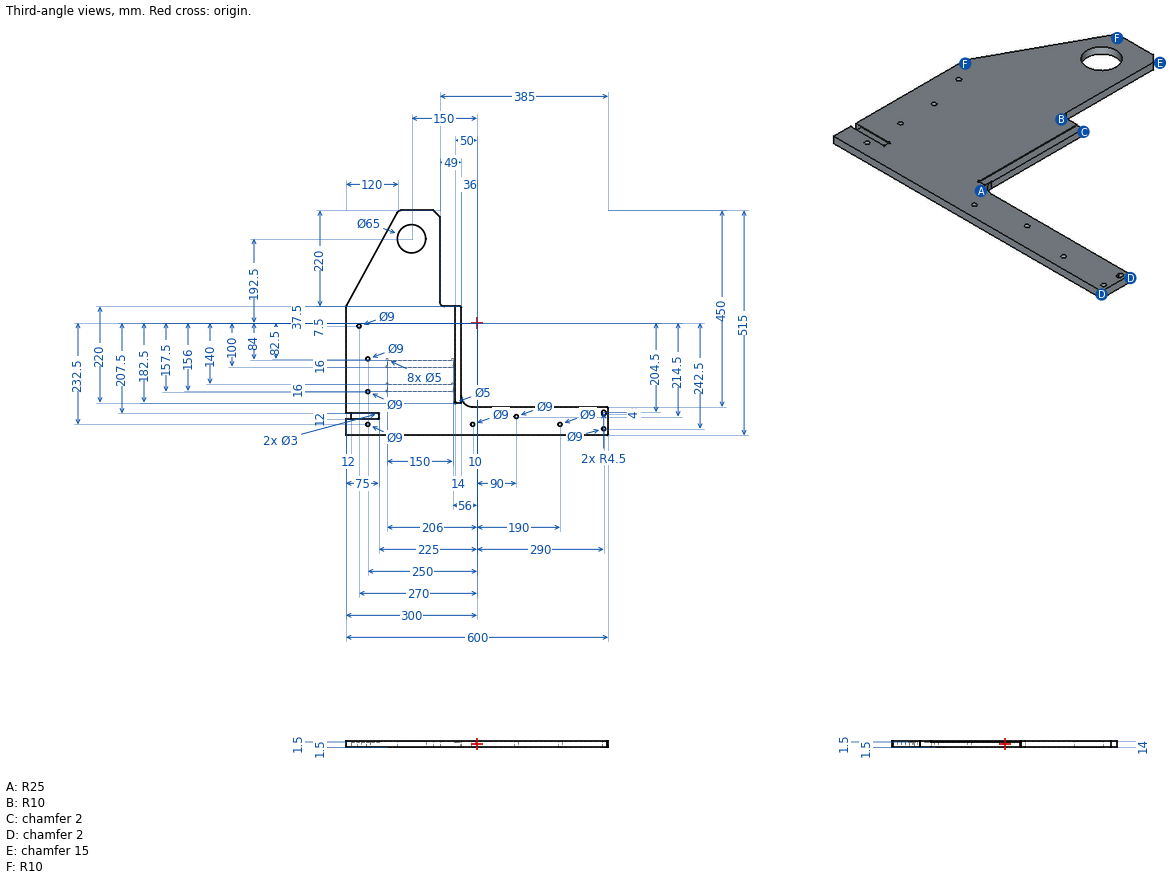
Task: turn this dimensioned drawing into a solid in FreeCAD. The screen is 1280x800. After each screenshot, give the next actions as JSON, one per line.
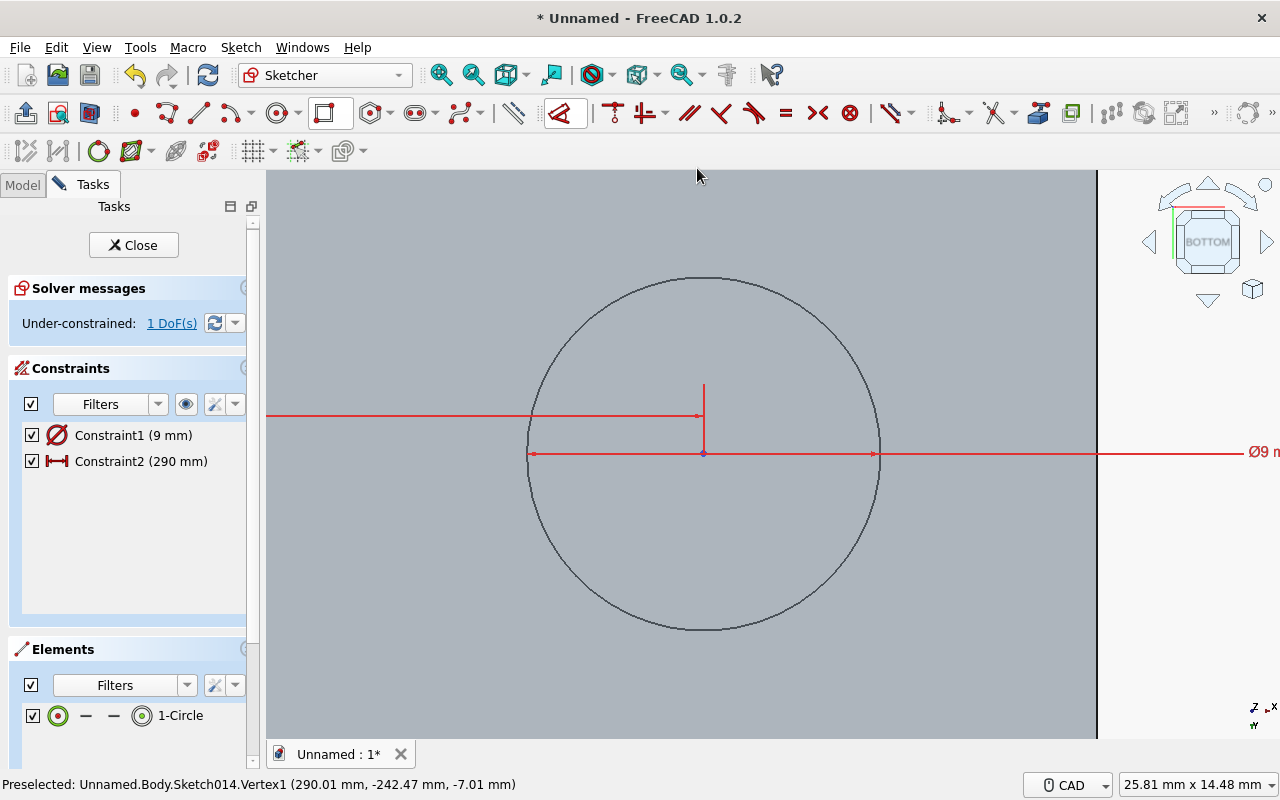
{"action": "left_click", "coordinate": [704, 454]}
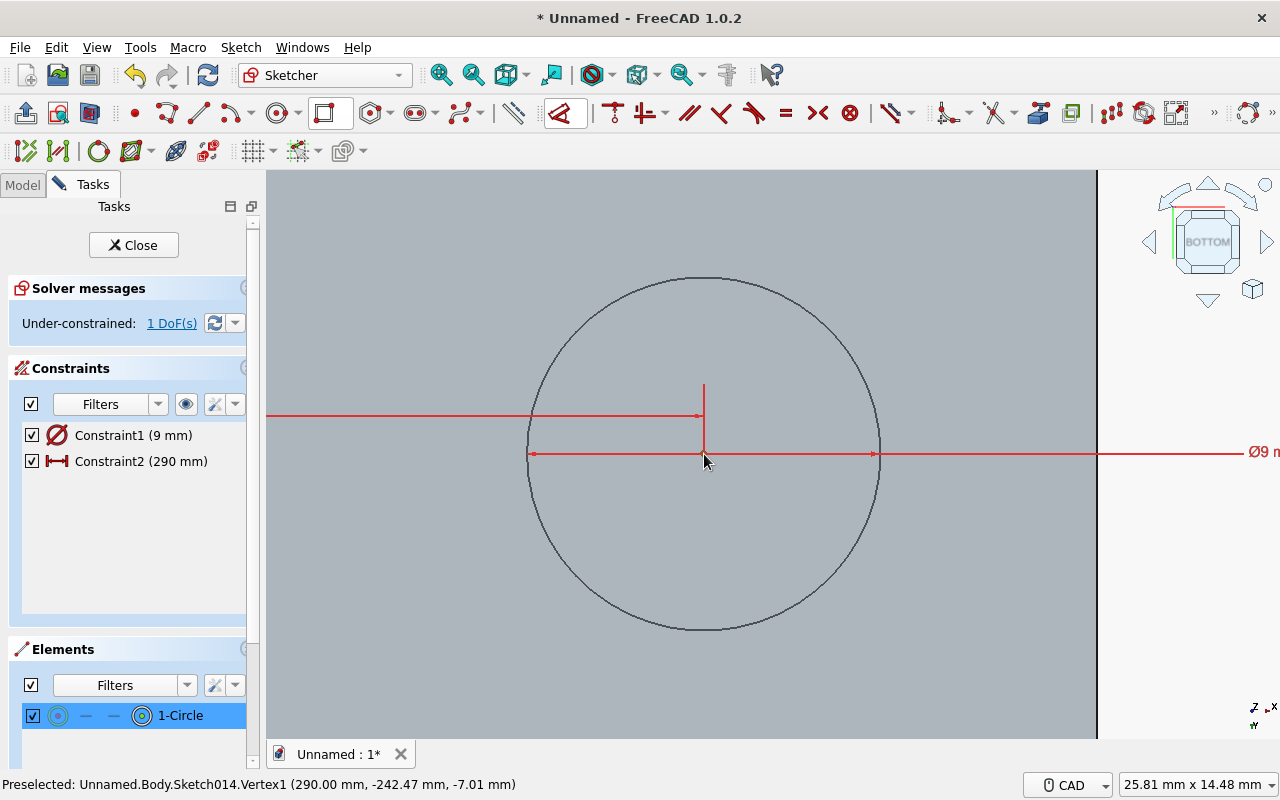
{"action": "left_click", "coordinate": [582, 114]}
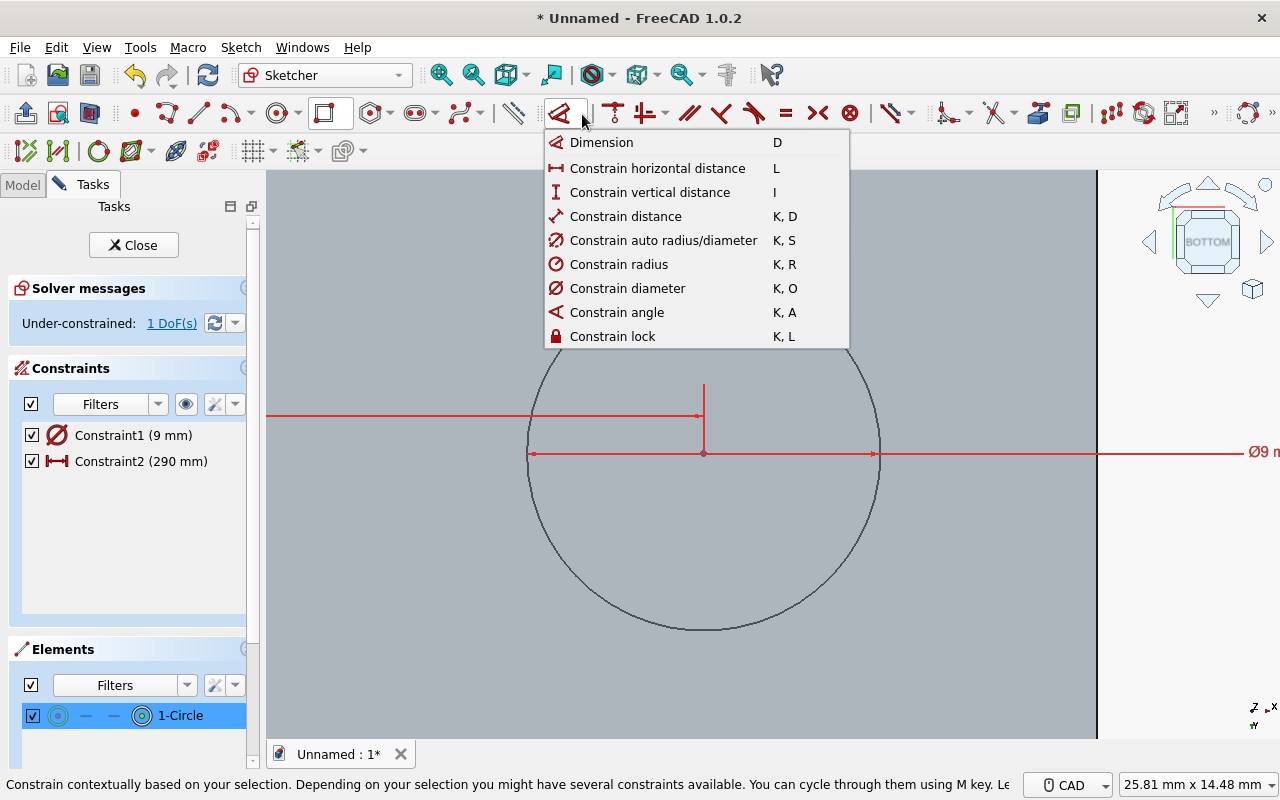
{"action": "left_click", "coordinate": [697, 192]}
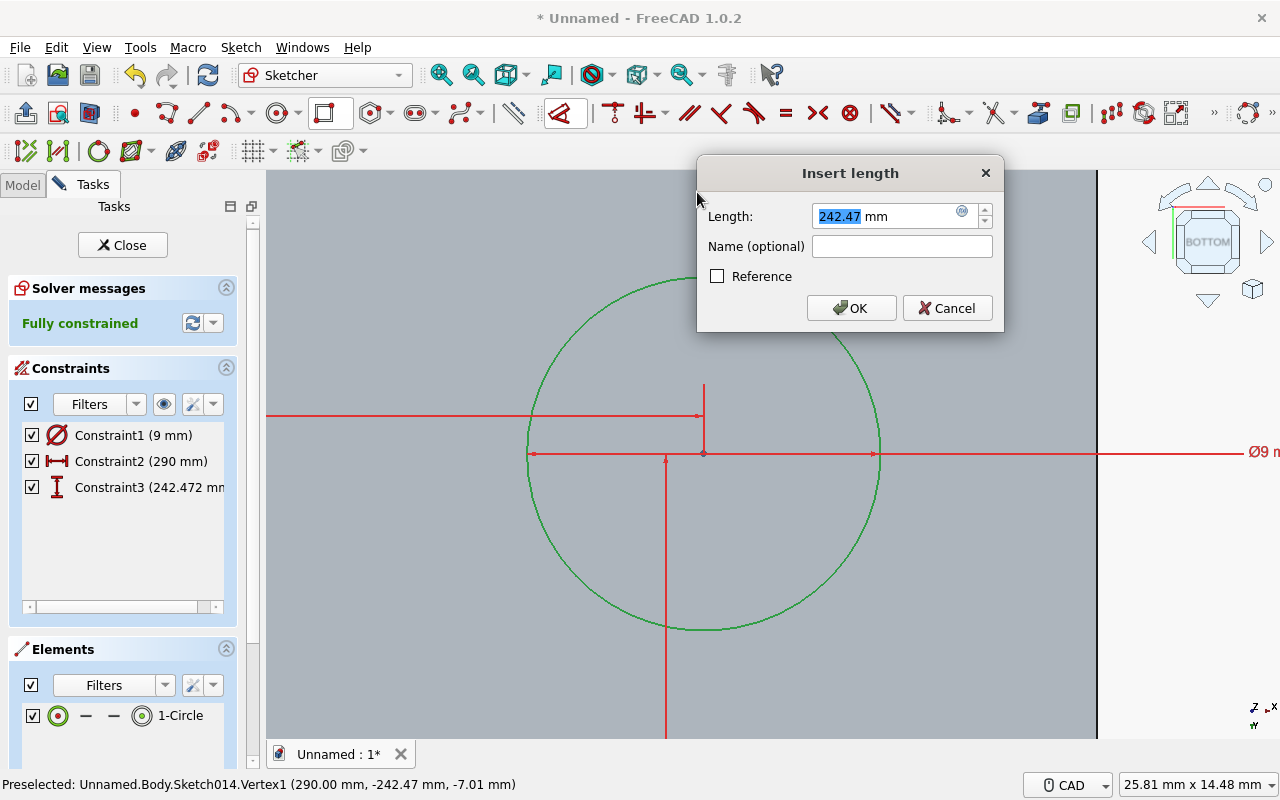
{"action": "type", "text": "242.5"}
{"action": "key", "text": "Return"}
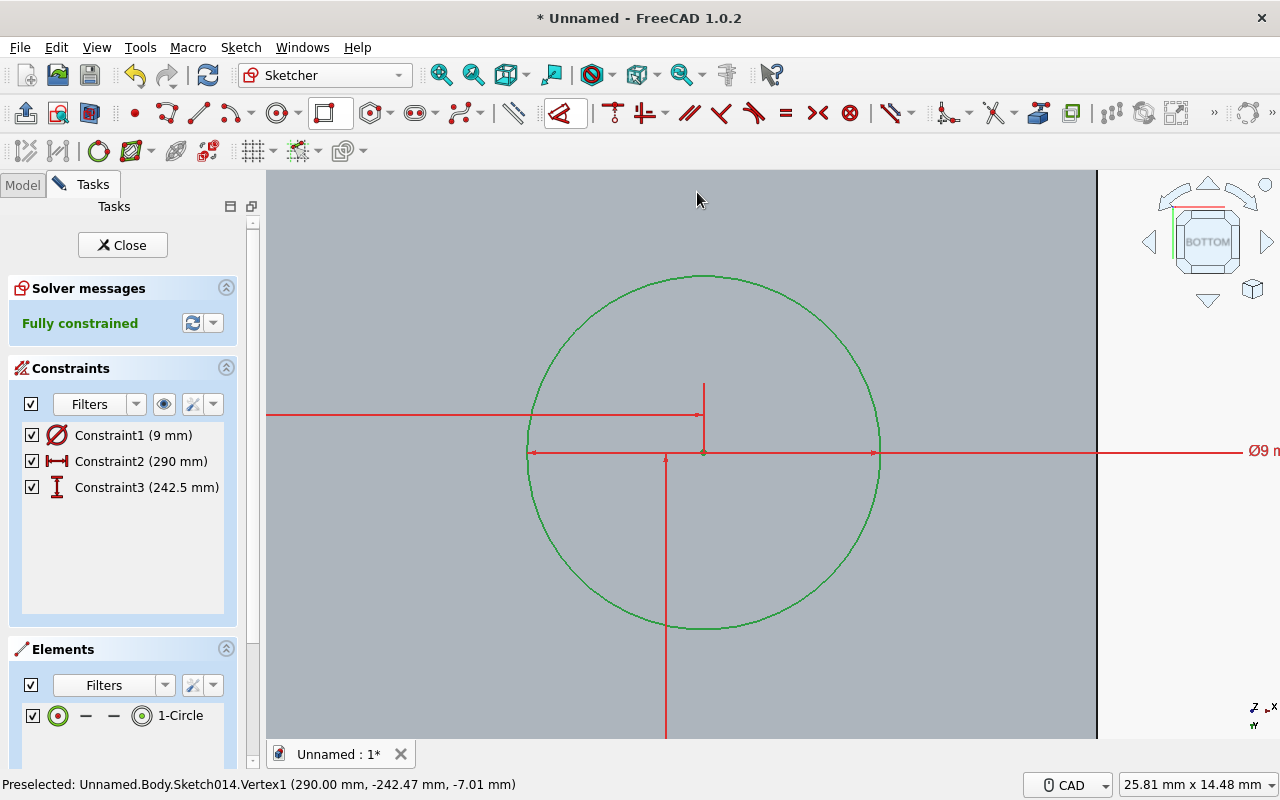
{"action": "left_click", "coordinate": [123, 245]}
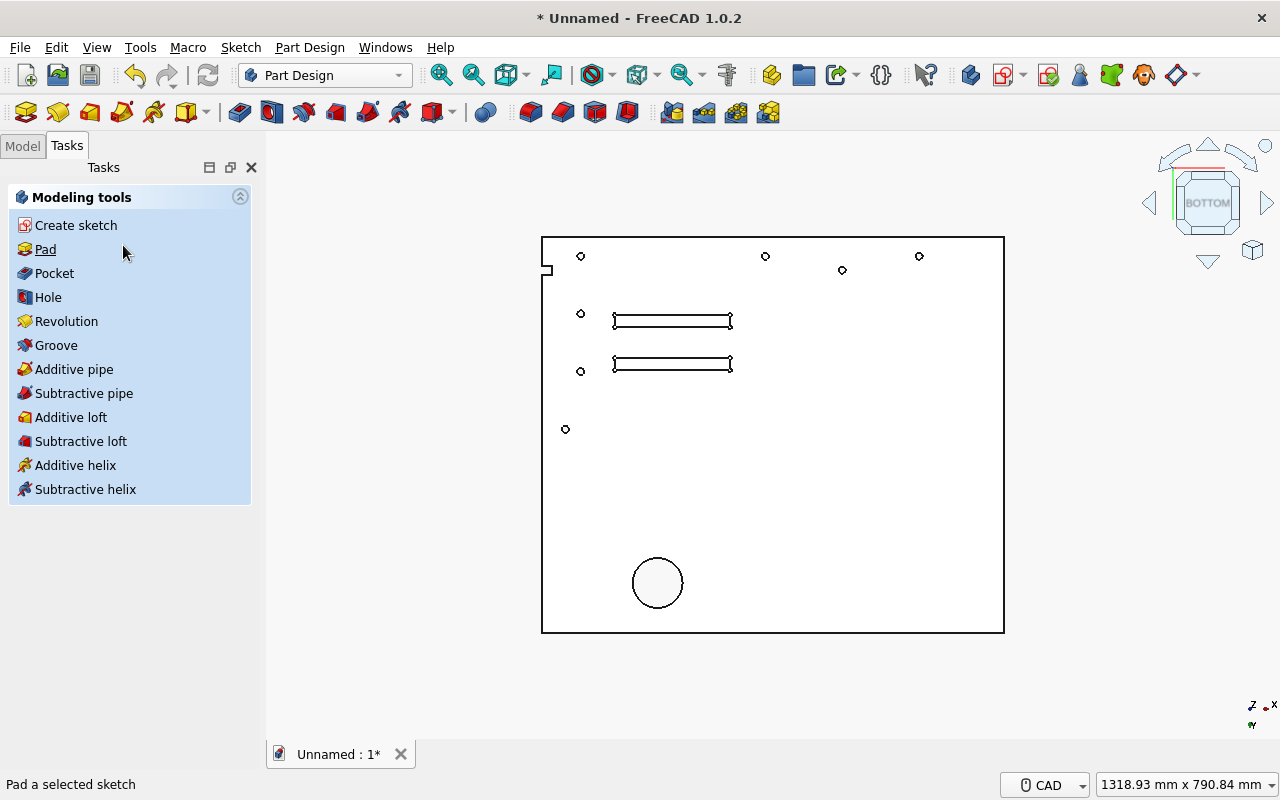
{"action": "left_click", "coordinate": [240, 112]}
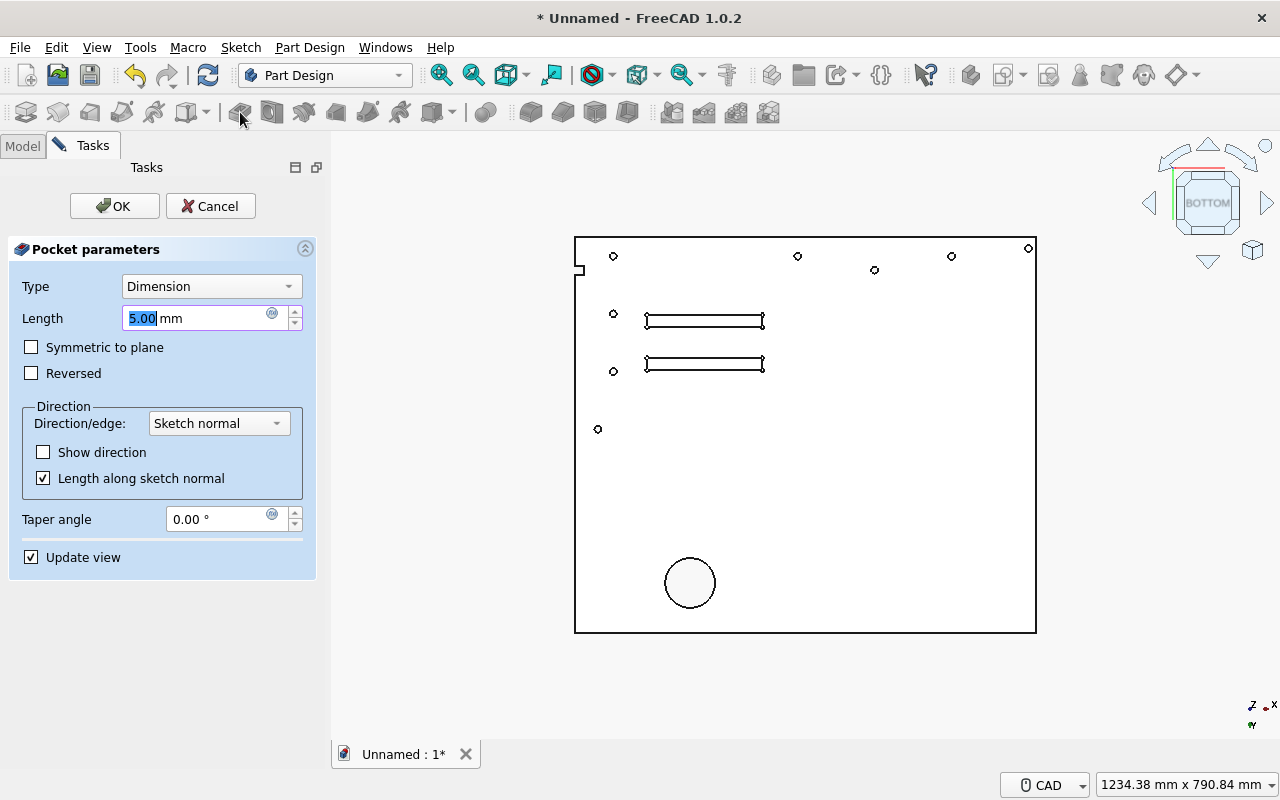
{"action": "left_click", "coordinate": [212, 286]}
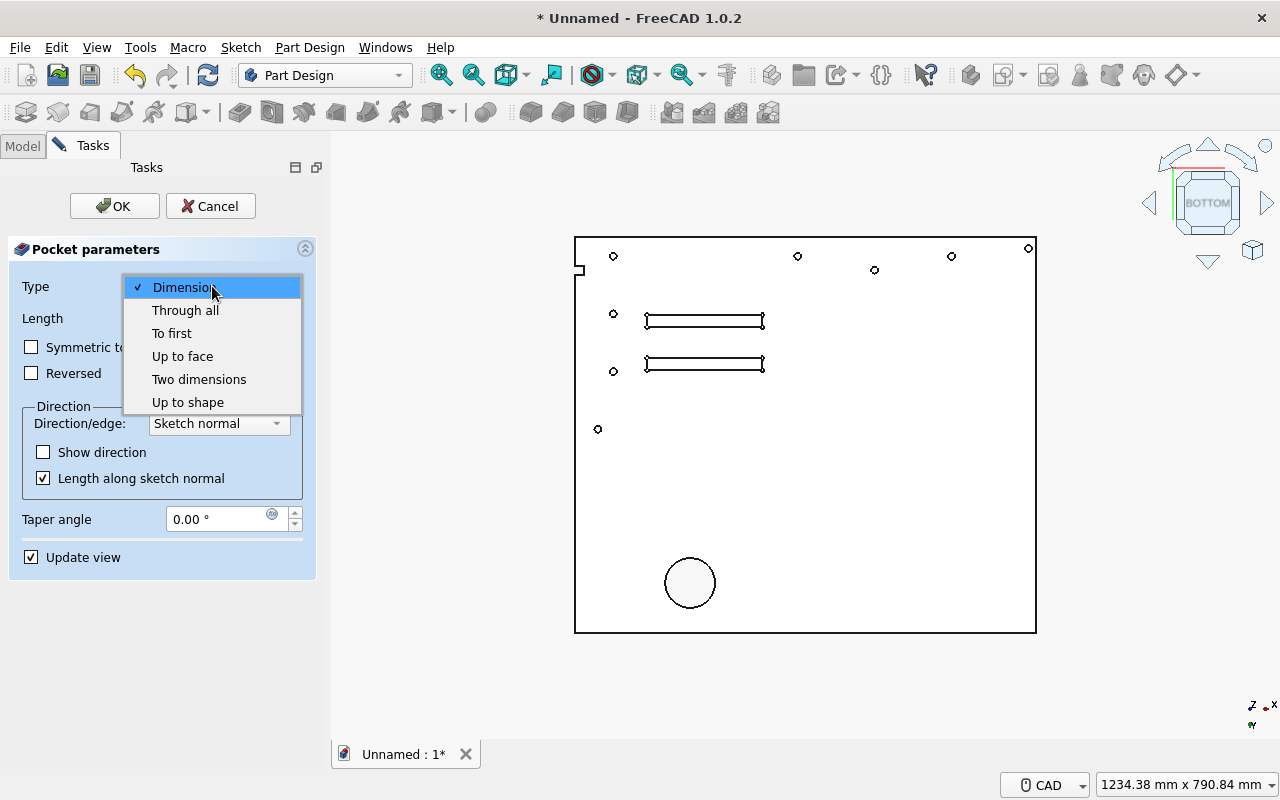
{"action": "left_click", "coordinate": [212, 334]}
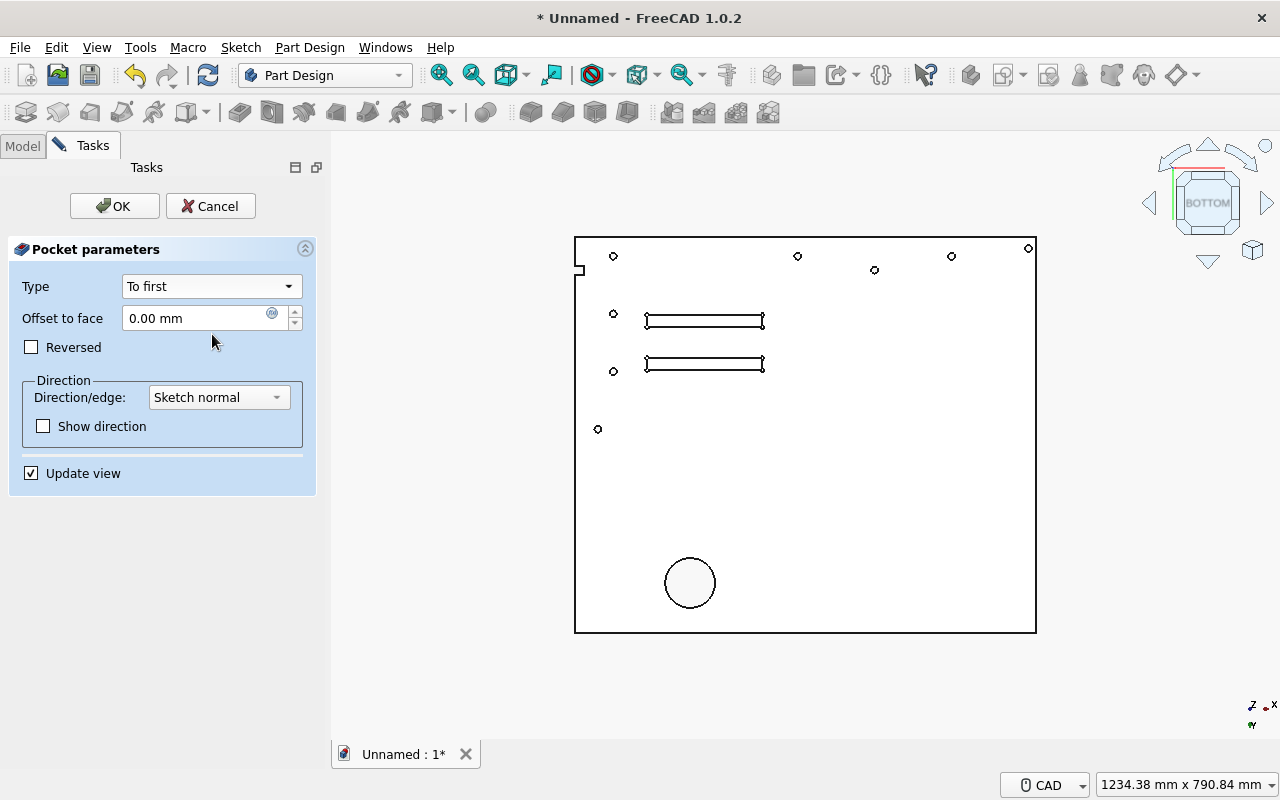
{"action": "left_click", "coordinate": [115, 206]}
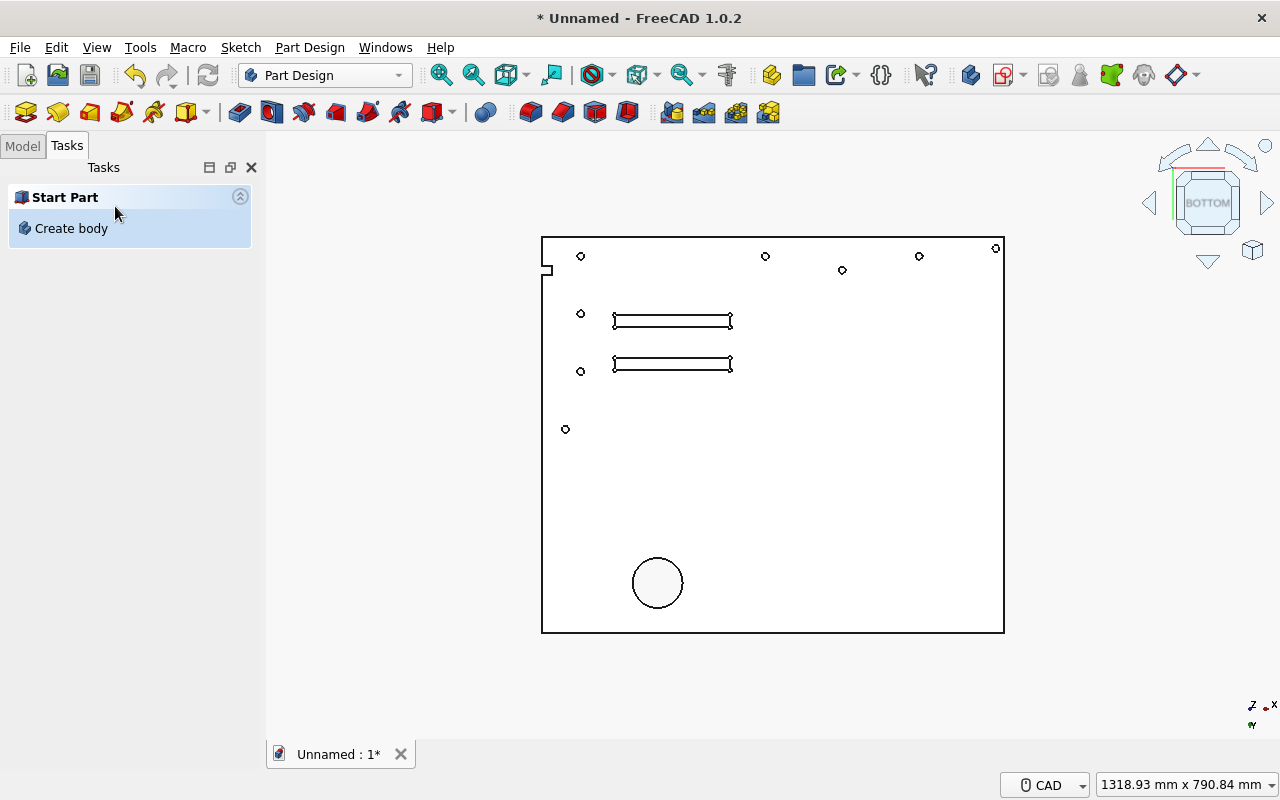
{"action": "left_click", "coordinate": [839, 491]}